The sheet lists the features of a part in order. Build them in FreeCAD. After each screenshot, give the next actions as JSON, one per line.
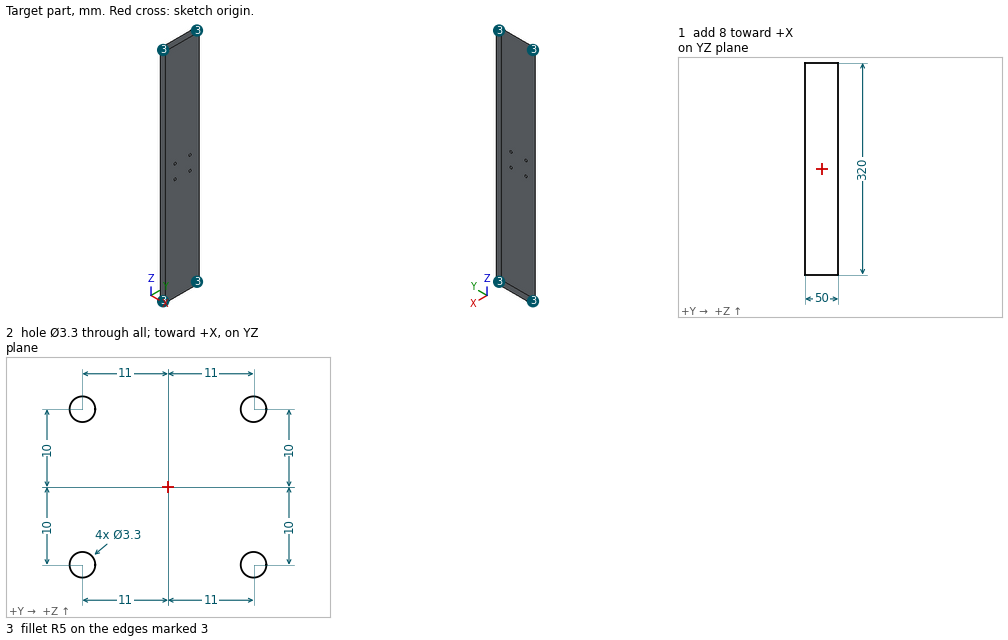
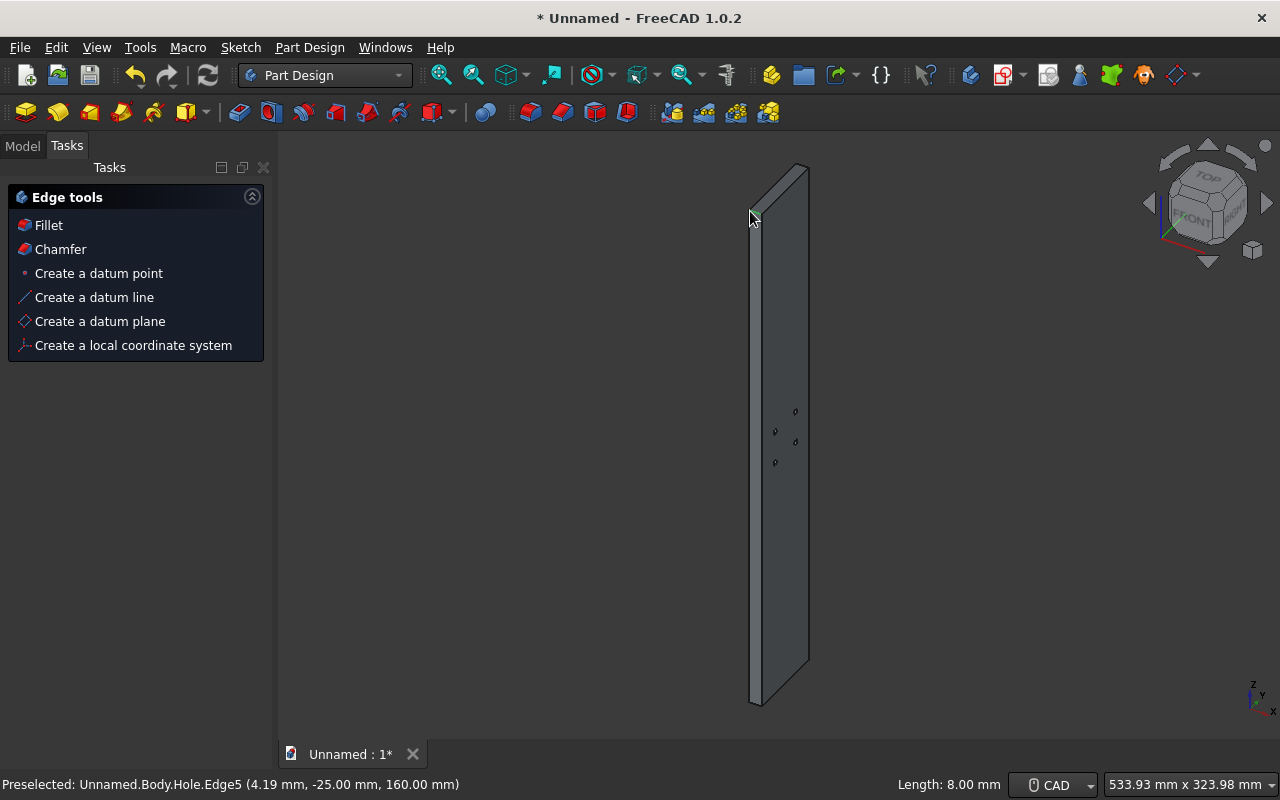
{"action": "scroll", "coordinate": [756, 703], "scroll_direction": "up", "scroll_amount": 5}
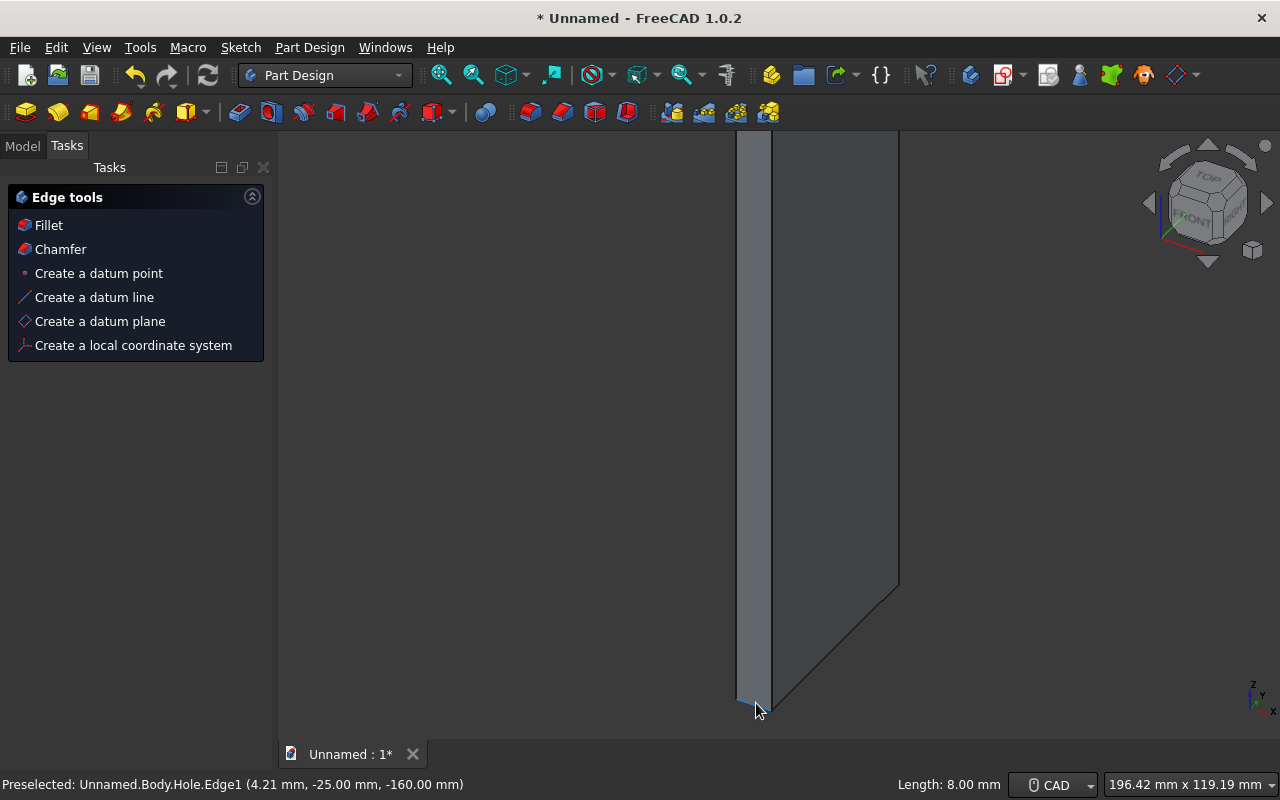
{"action": "left_click", "coordinate": [442, 76]}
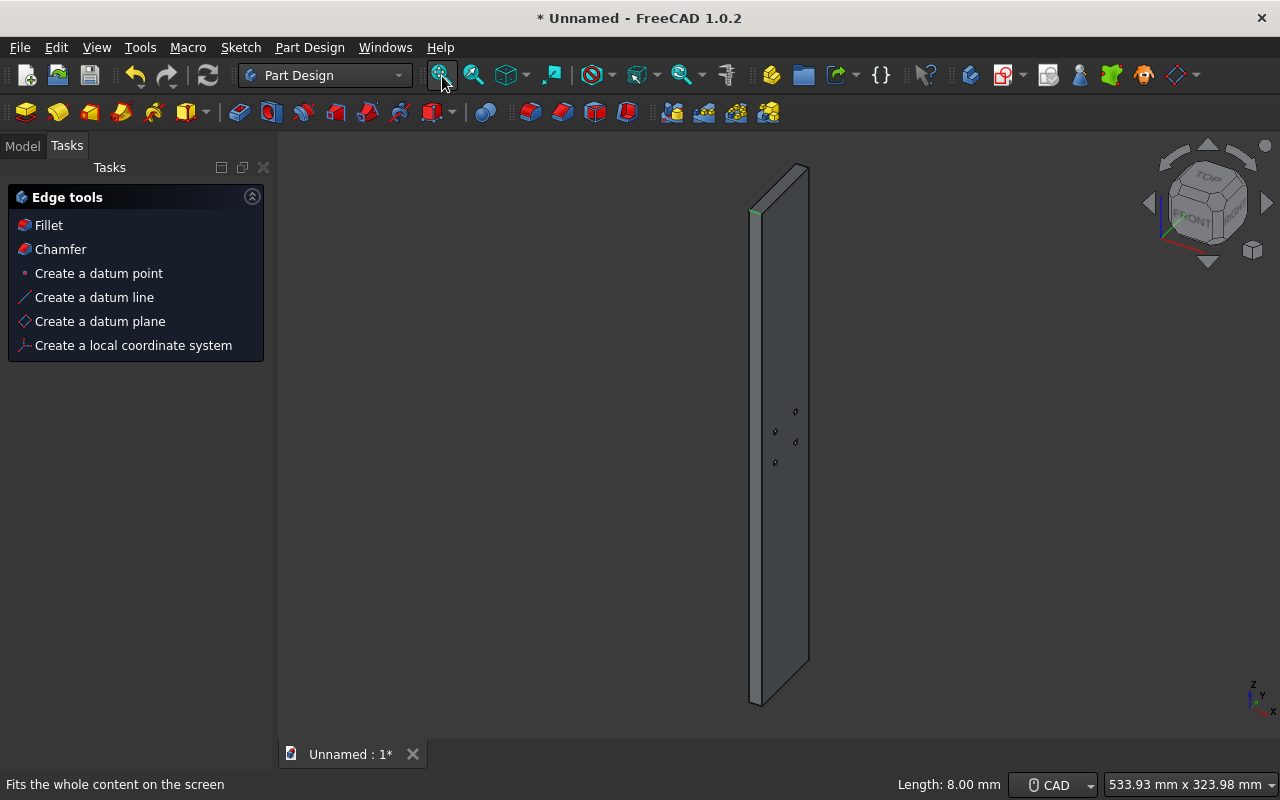
{"action": "key", "text": "0"}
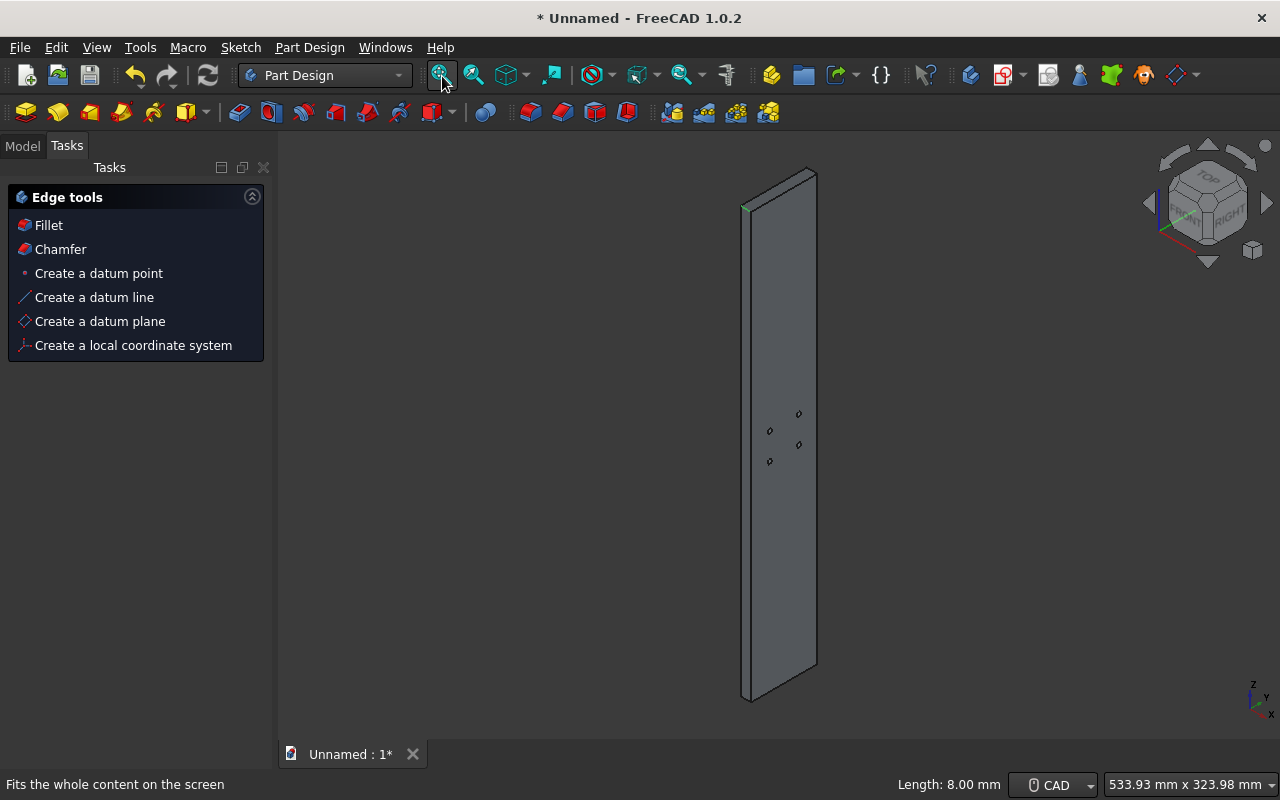
{"action": "scroll", "coordinate": [746, 698], "scroll_direction": "up", "scroll_amount": 5}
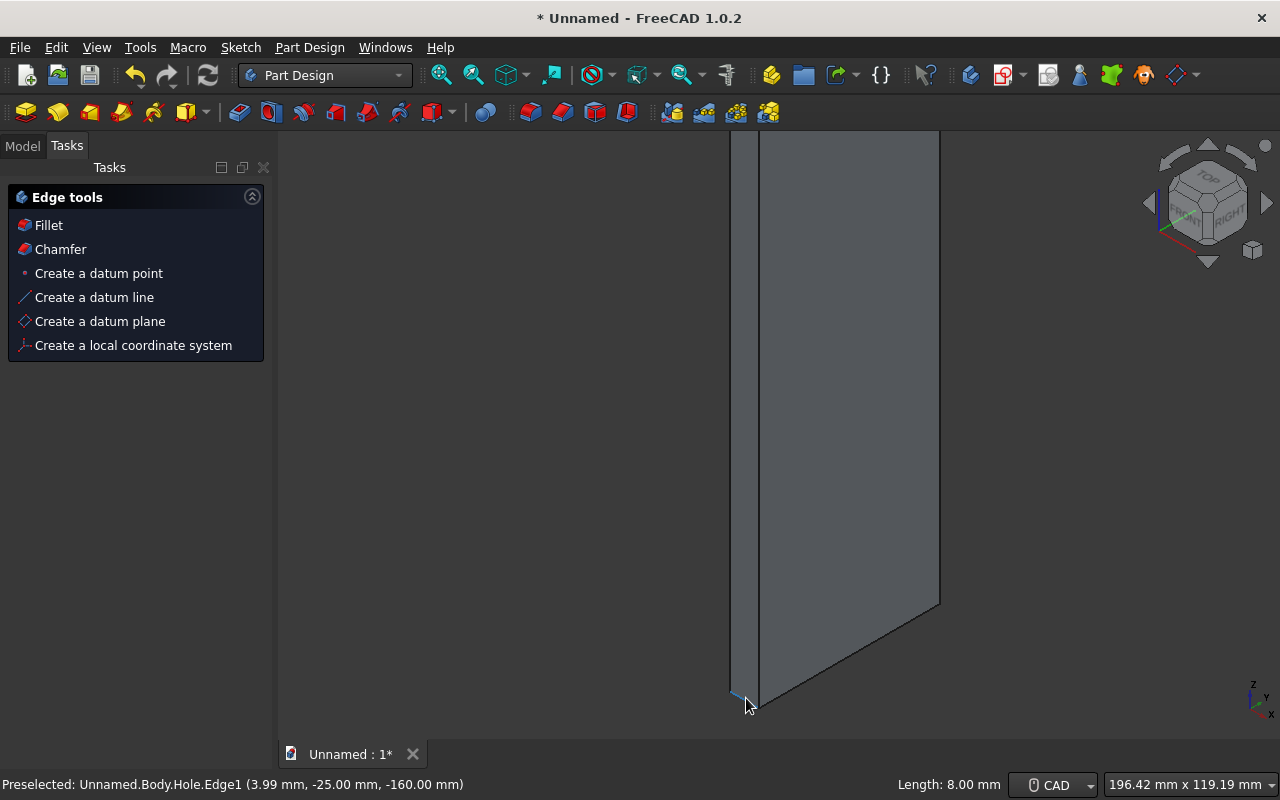
{"action": "key", "text": "v f"}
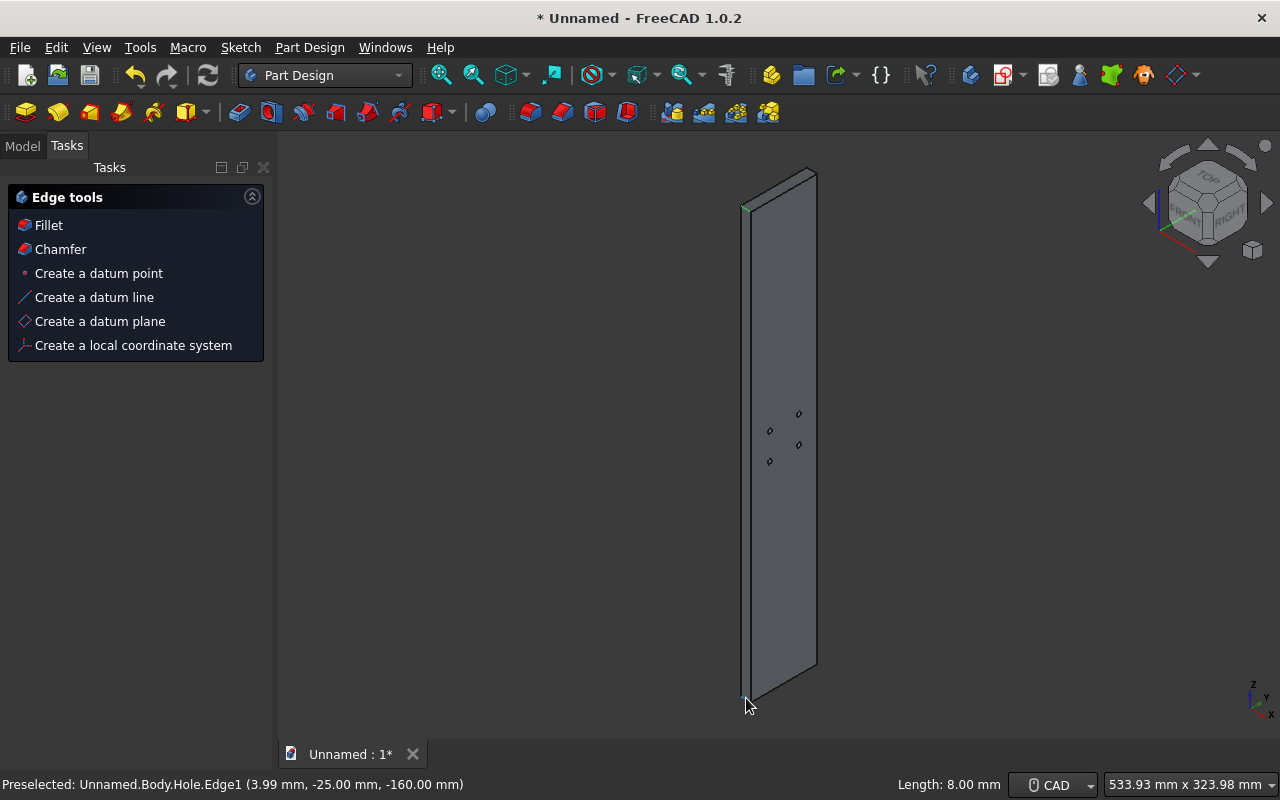
{"action": "key", "text": "2"}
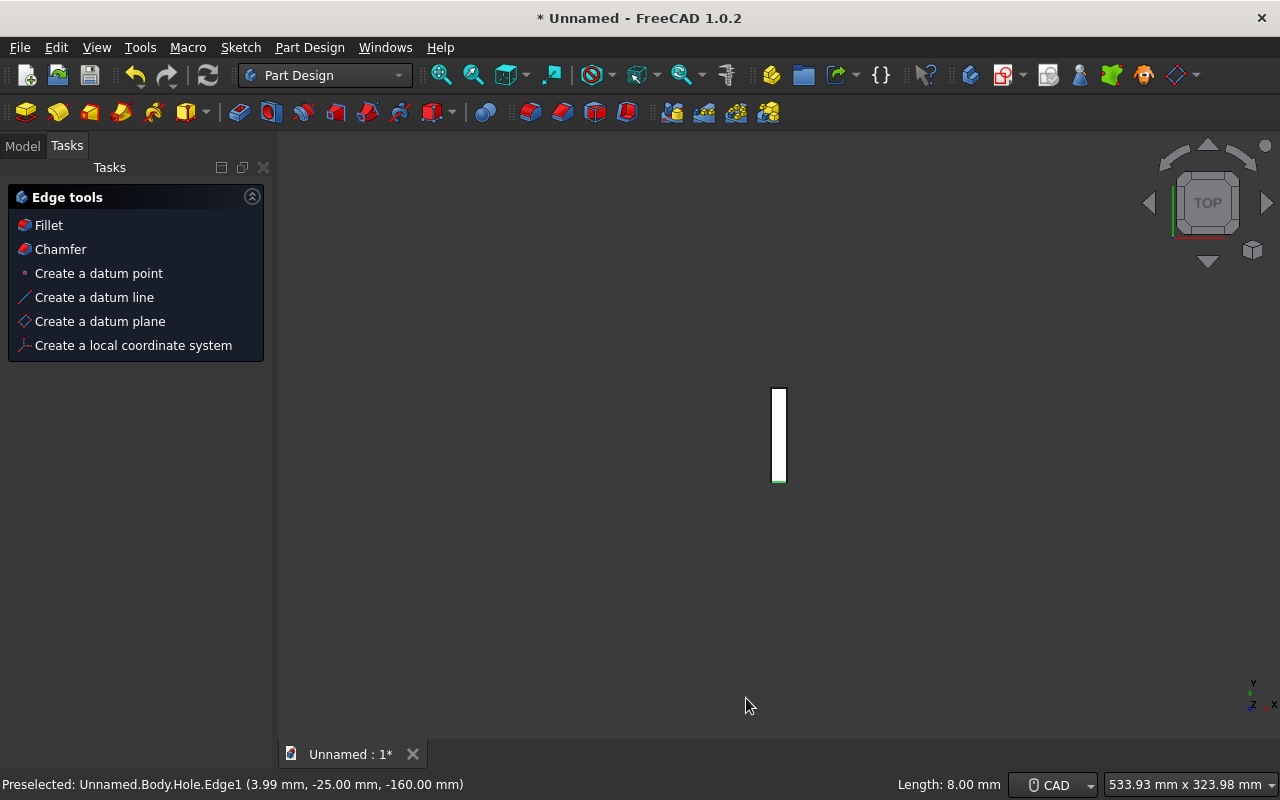
{"action": "left_click", "coordinate": [442, 76]}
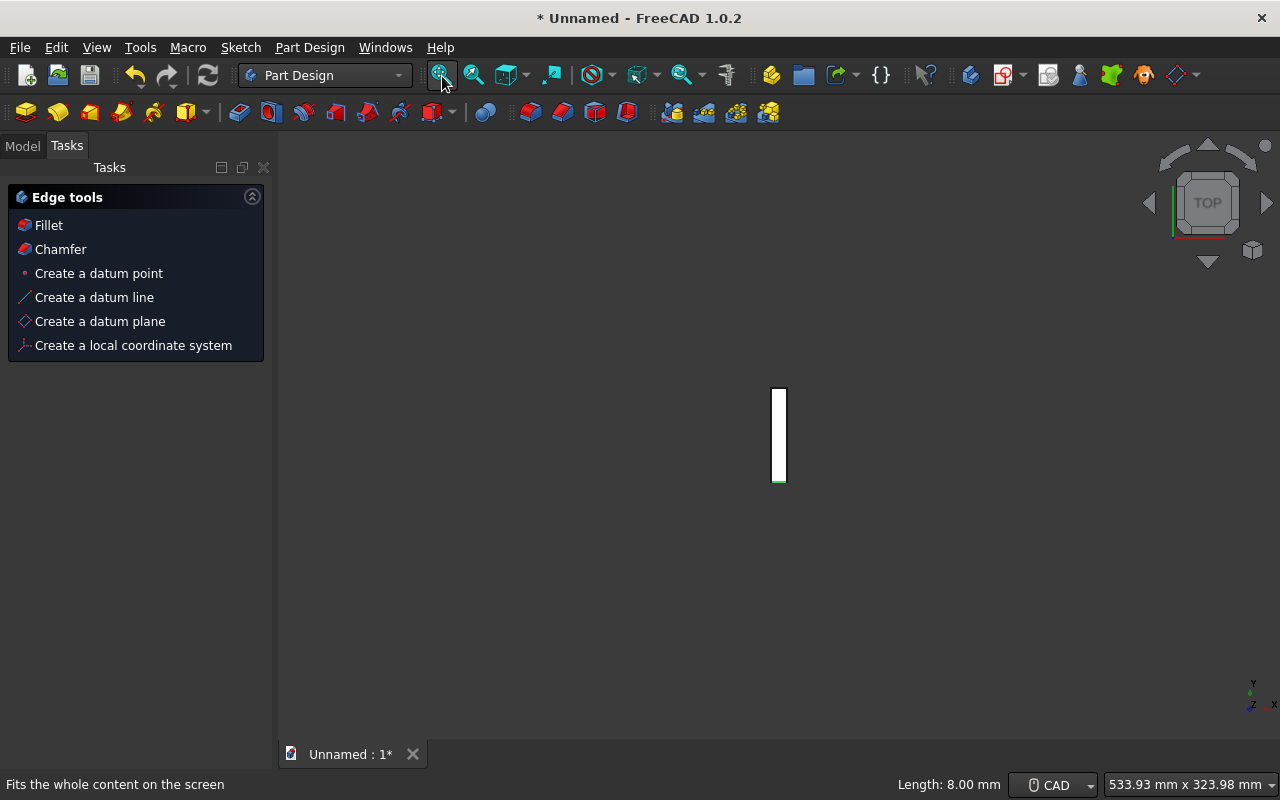
{"action": "left_click", "coordinate": [779, 387], "text": "ctrl"}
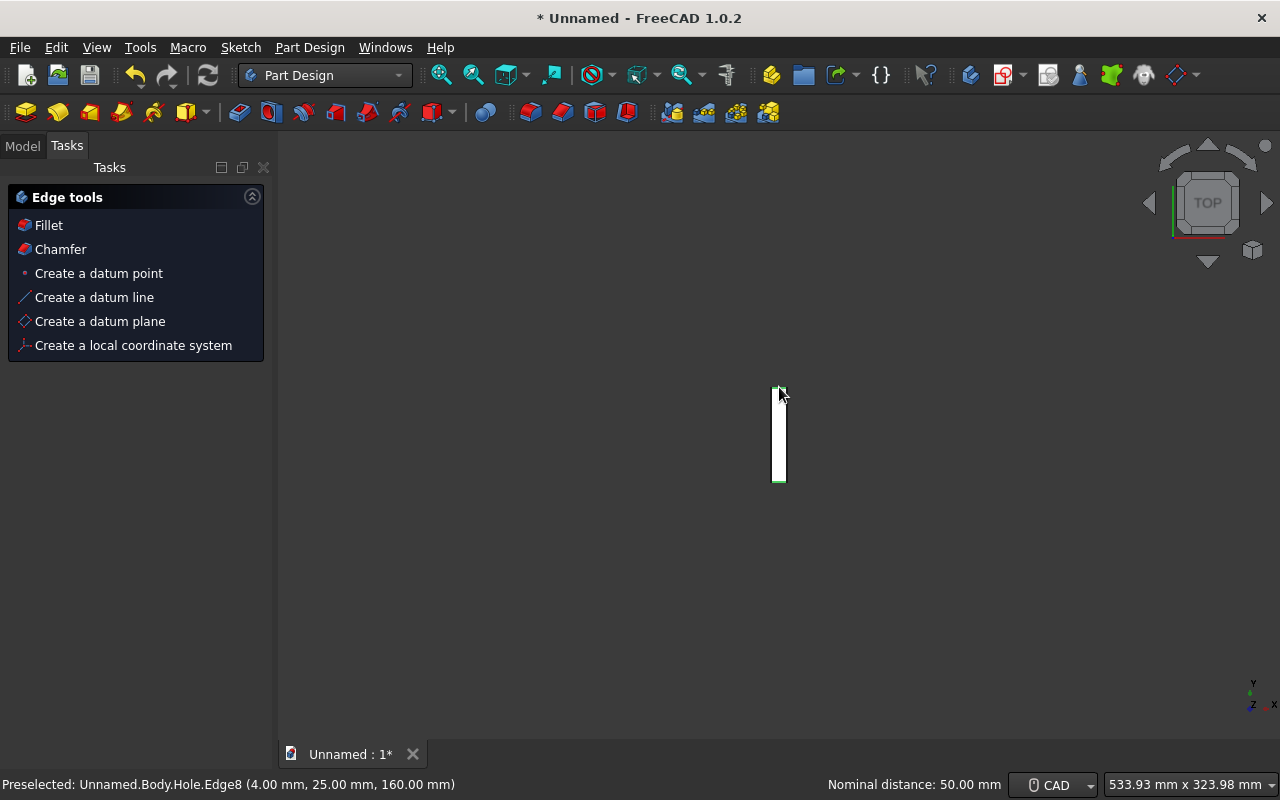
{"action": "scroll", "coordinate": [779, 481], "scroll_direction": "up", "scroll_amount": 5}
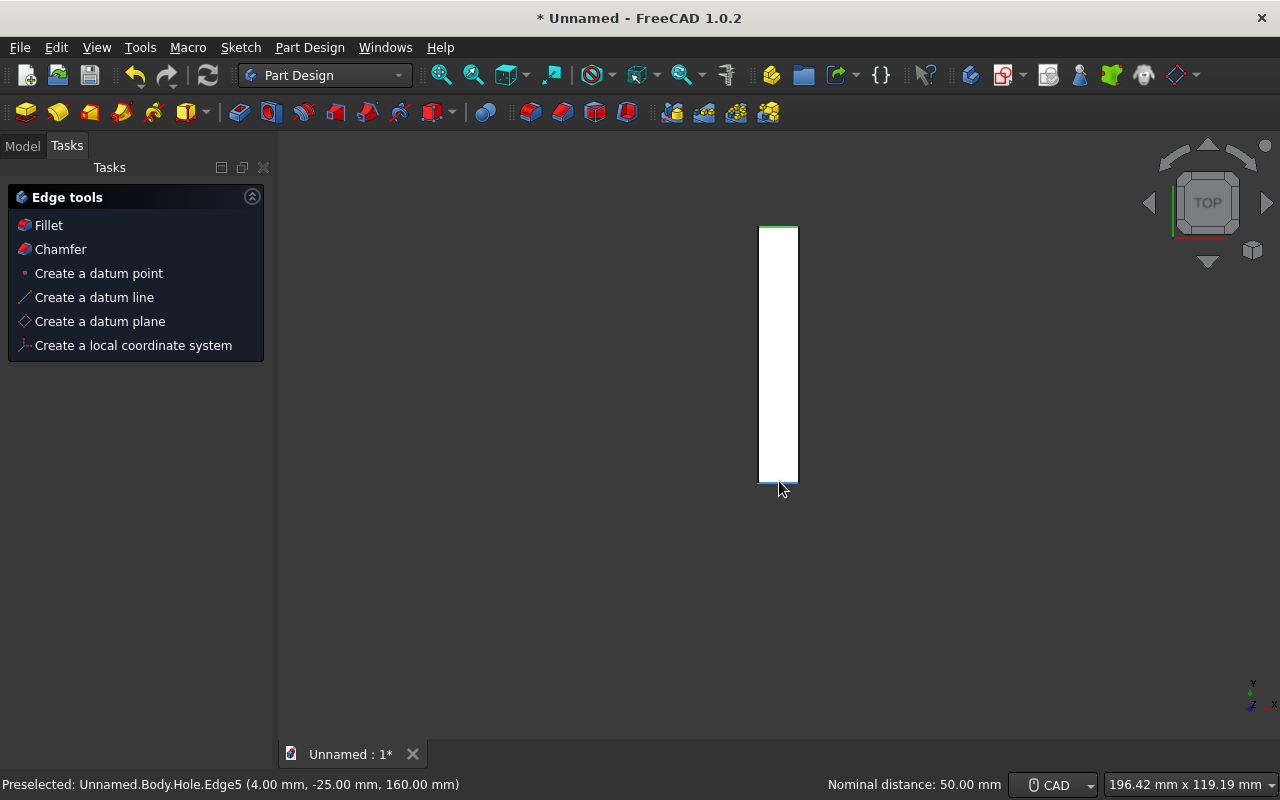
{"action": "key", "text": "v f"}